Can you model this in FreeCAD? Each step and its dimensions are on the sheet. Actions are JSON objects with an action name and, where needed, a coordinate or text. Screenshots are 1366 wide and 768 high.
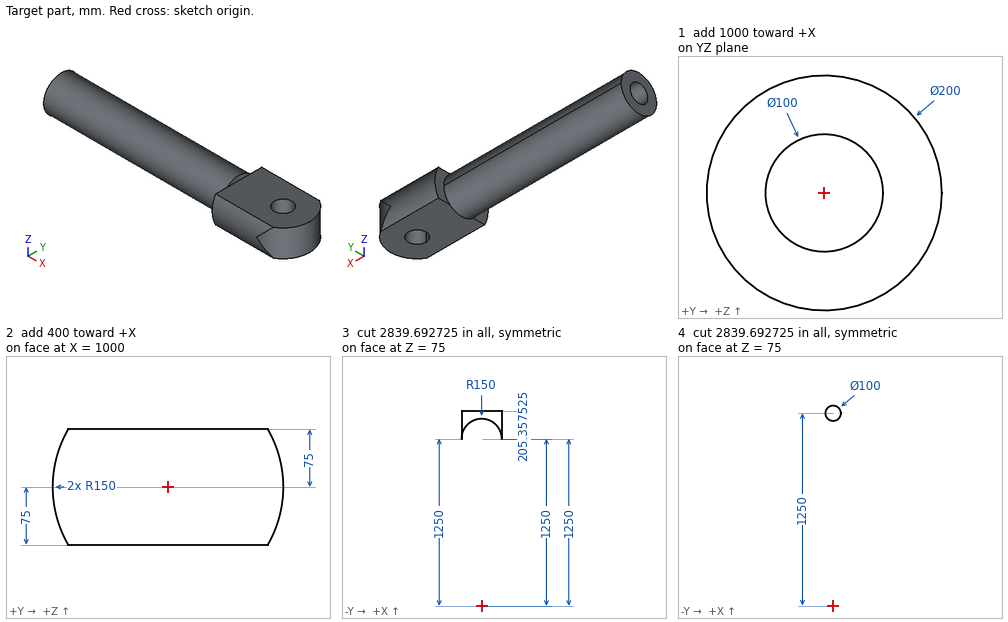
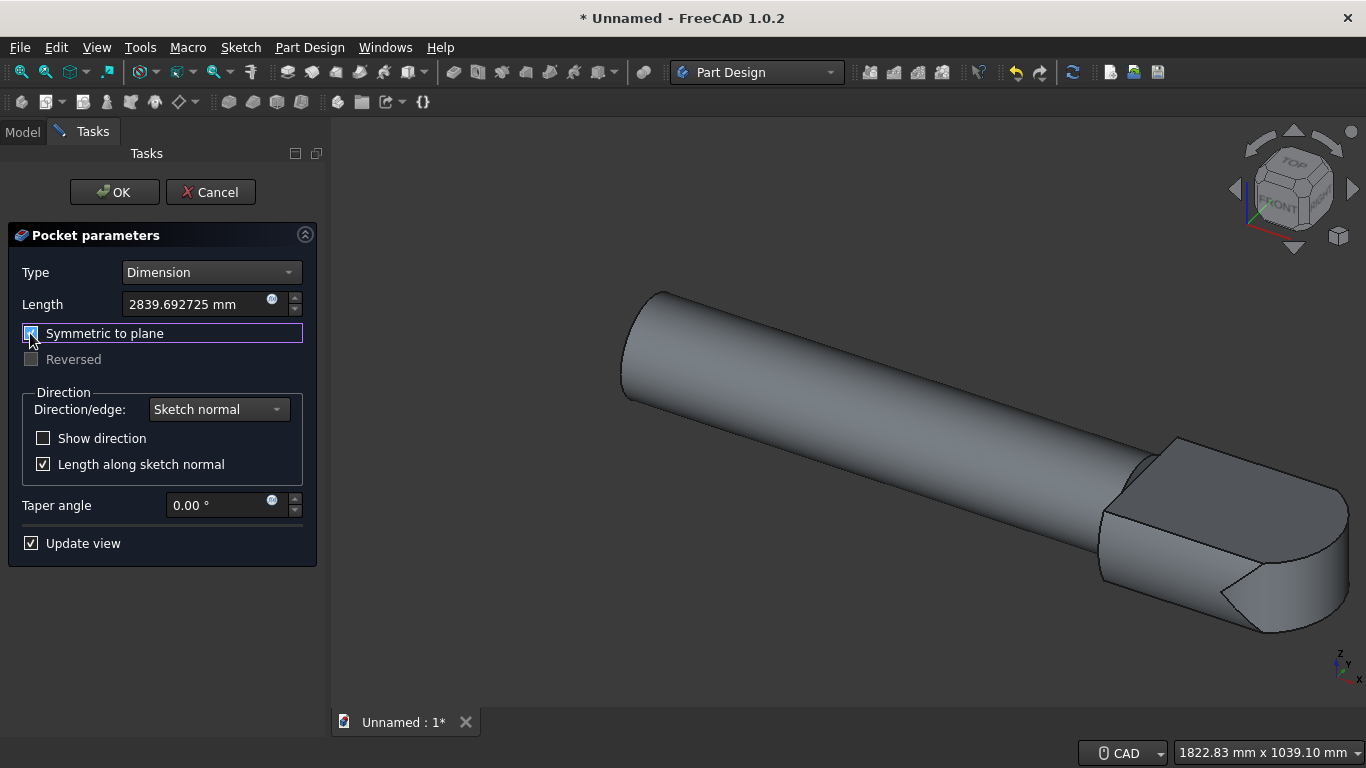
{"action": "left_click", "coordinate": [115, 192]}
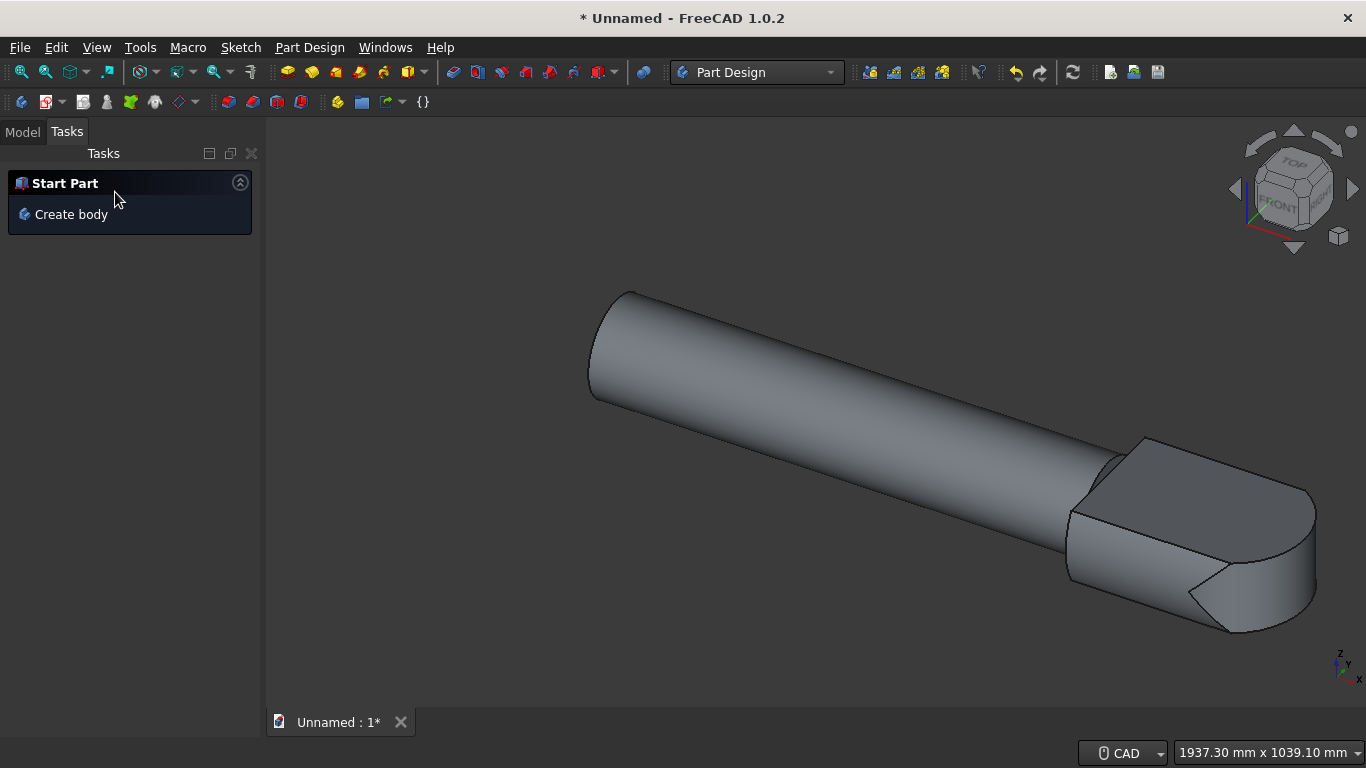
{"action": "left_click", "coordinate": [1207, 506]}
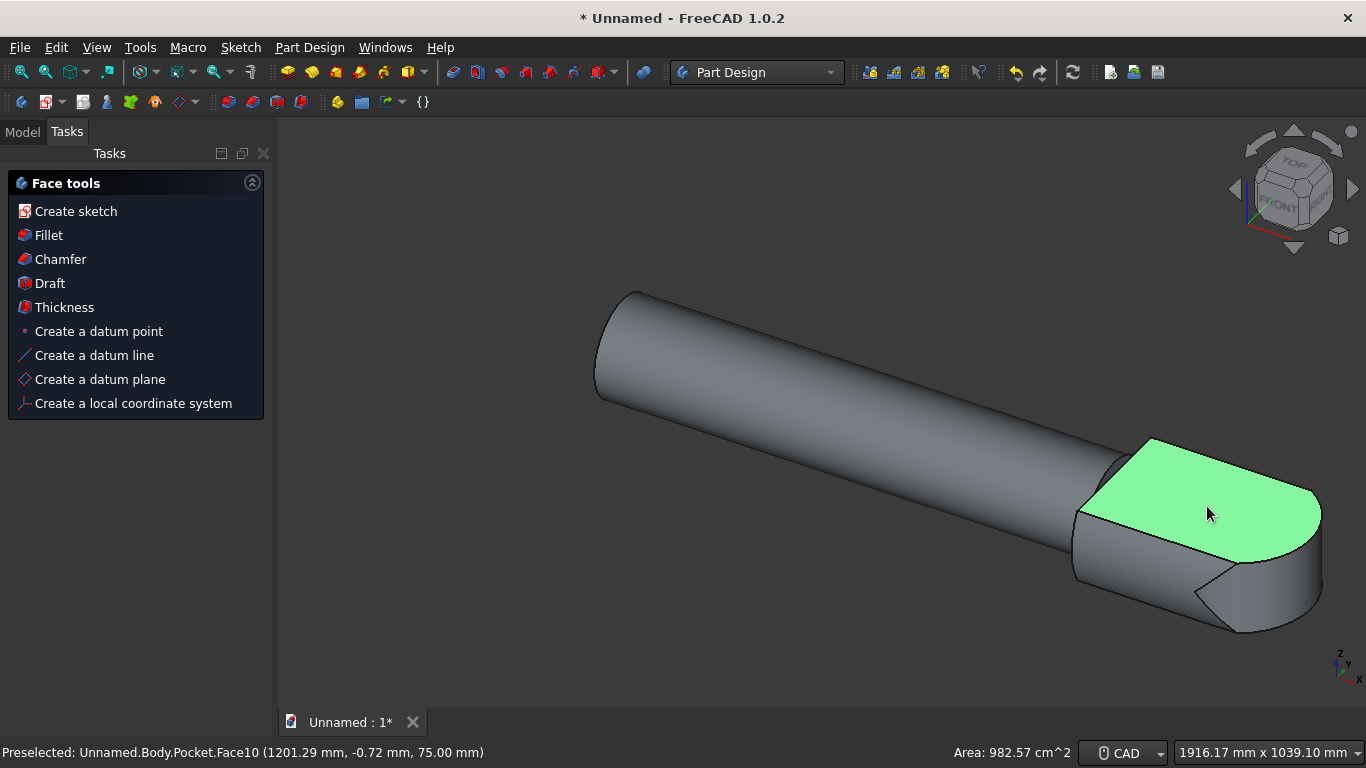
{"action": "left_click", "coordinate": [46, 102]}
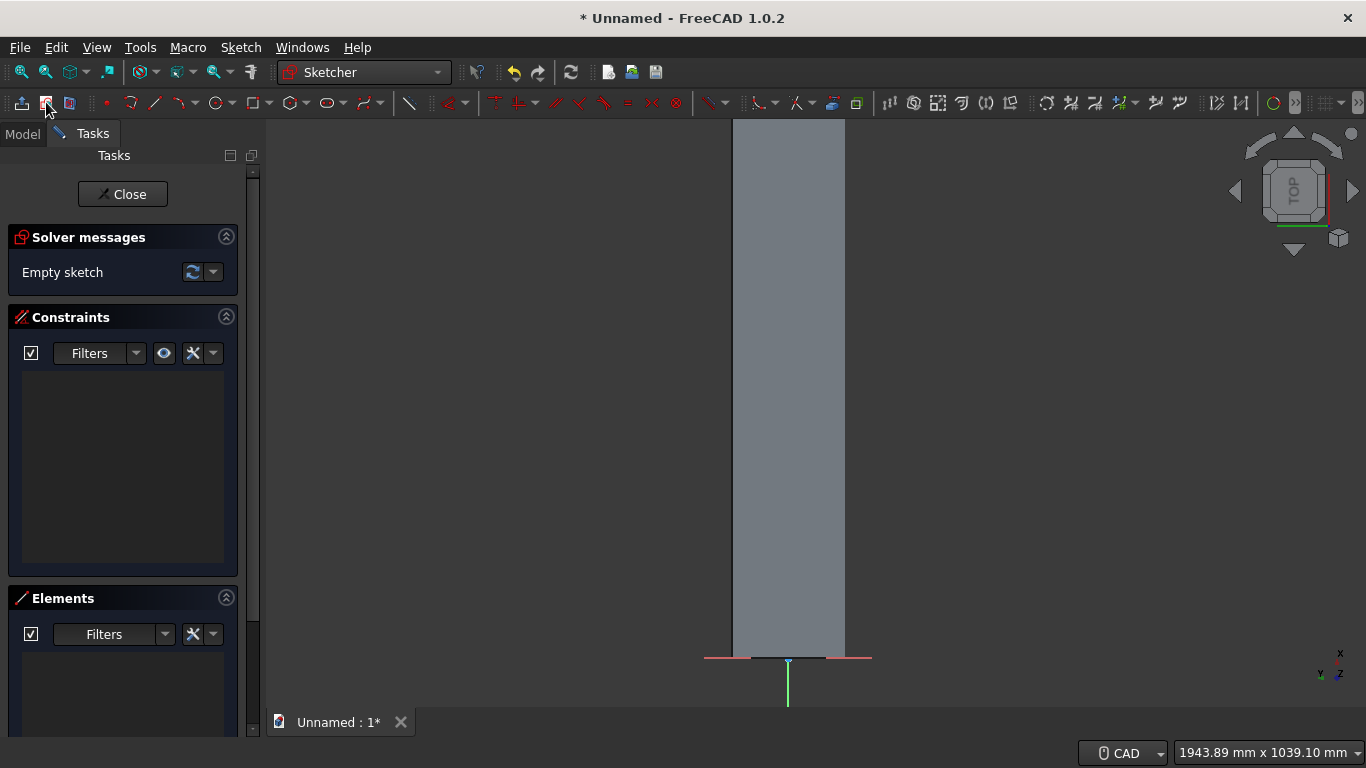
{"action": "left_click", "coordinate": [70, 104]}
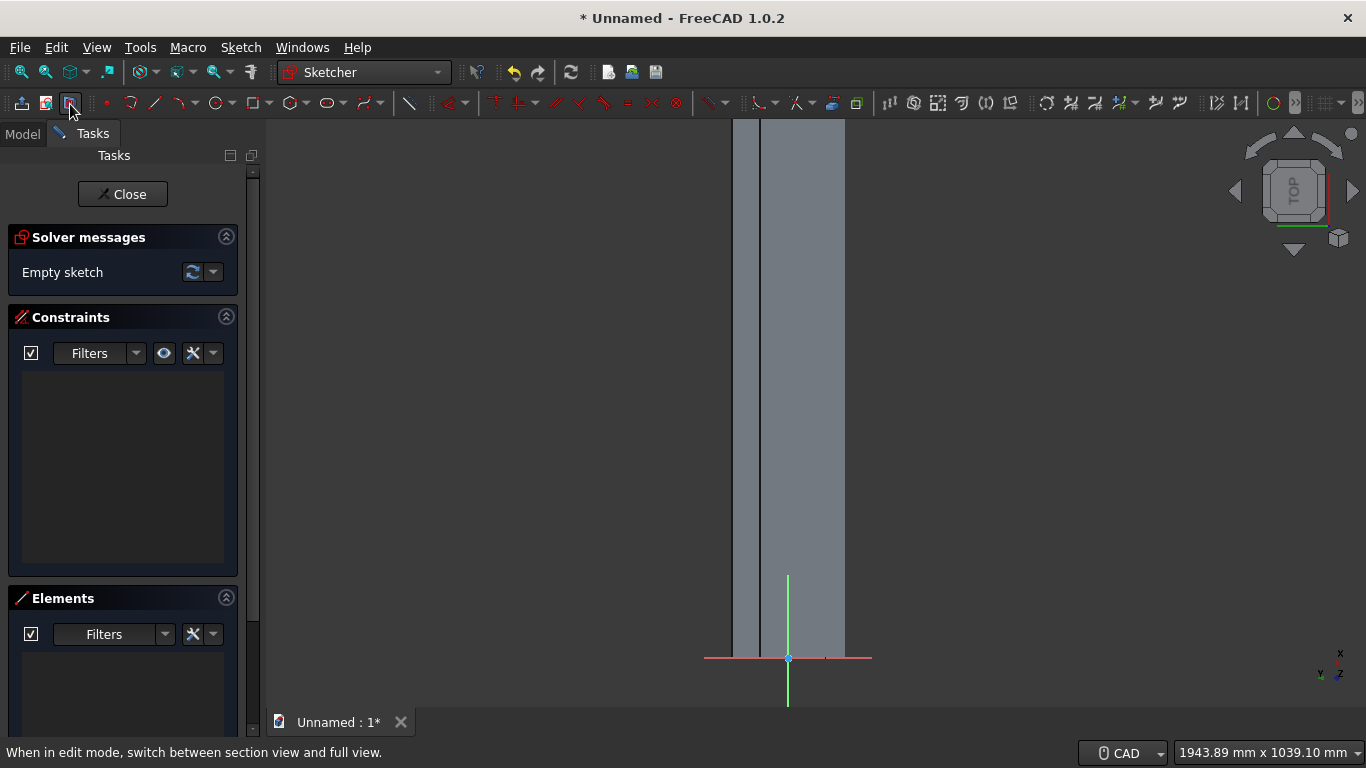
{"action": "scroll", "coordinate": [748, 413], "scroll_direction": "down", "scroll_amount": 5}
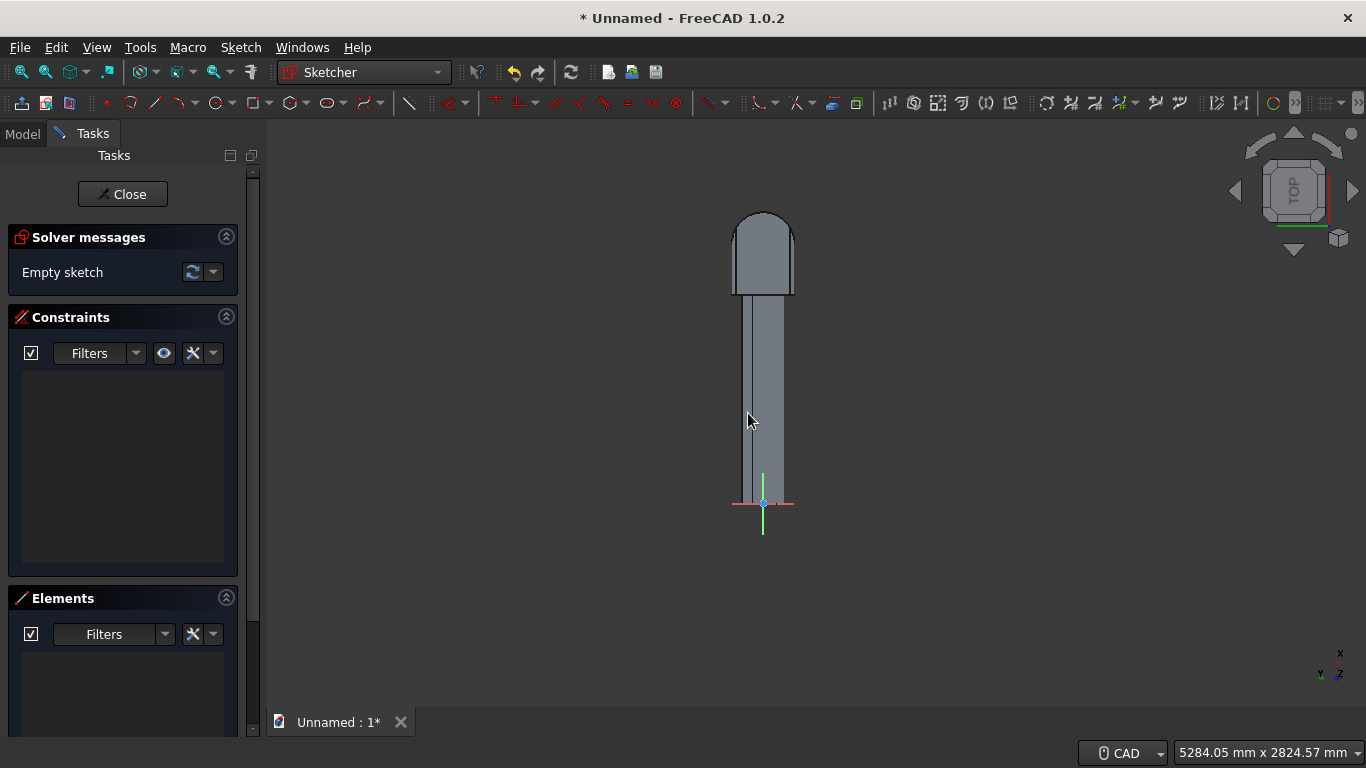
{"action": "scroll", "coordinate": [764, 232], "scroll_direction": "up", "scroll_amount": 14}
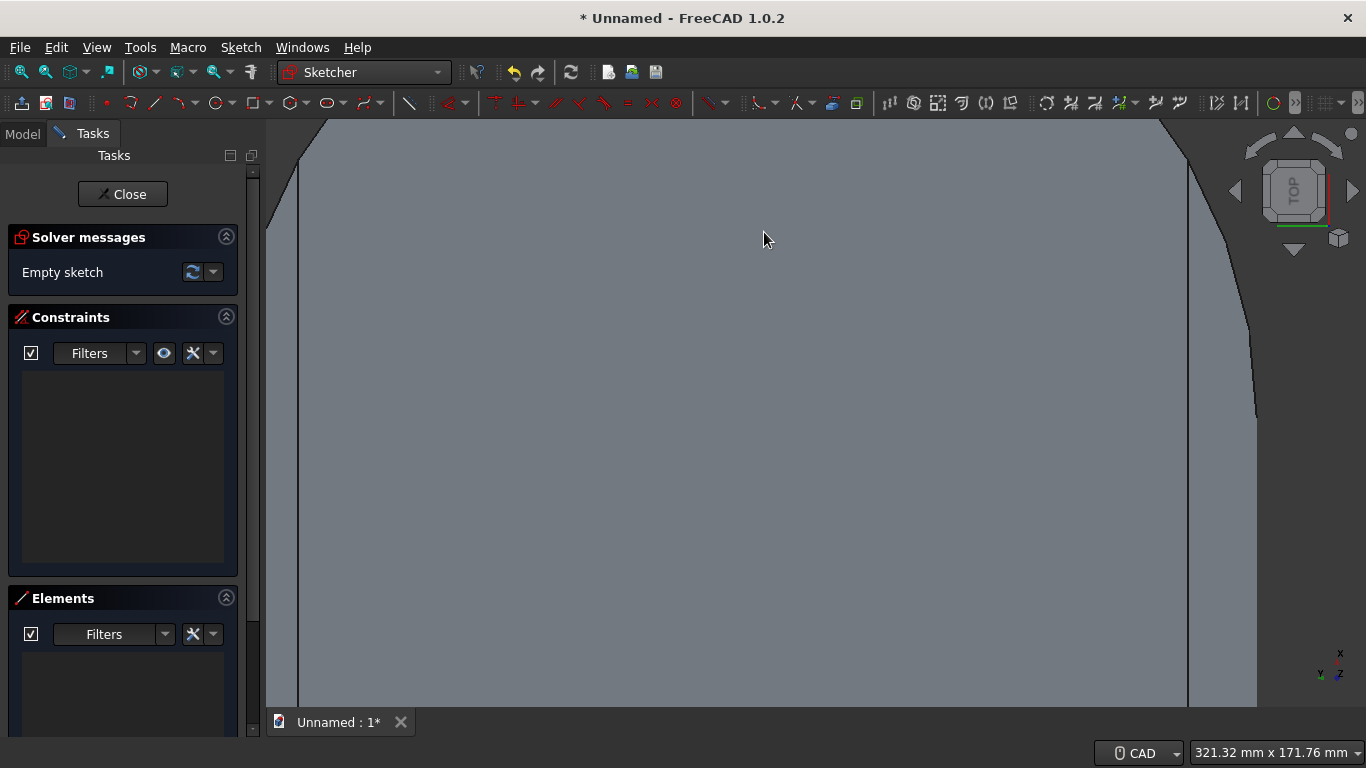
{"action": "left_click", "coordinate": [216, 104]}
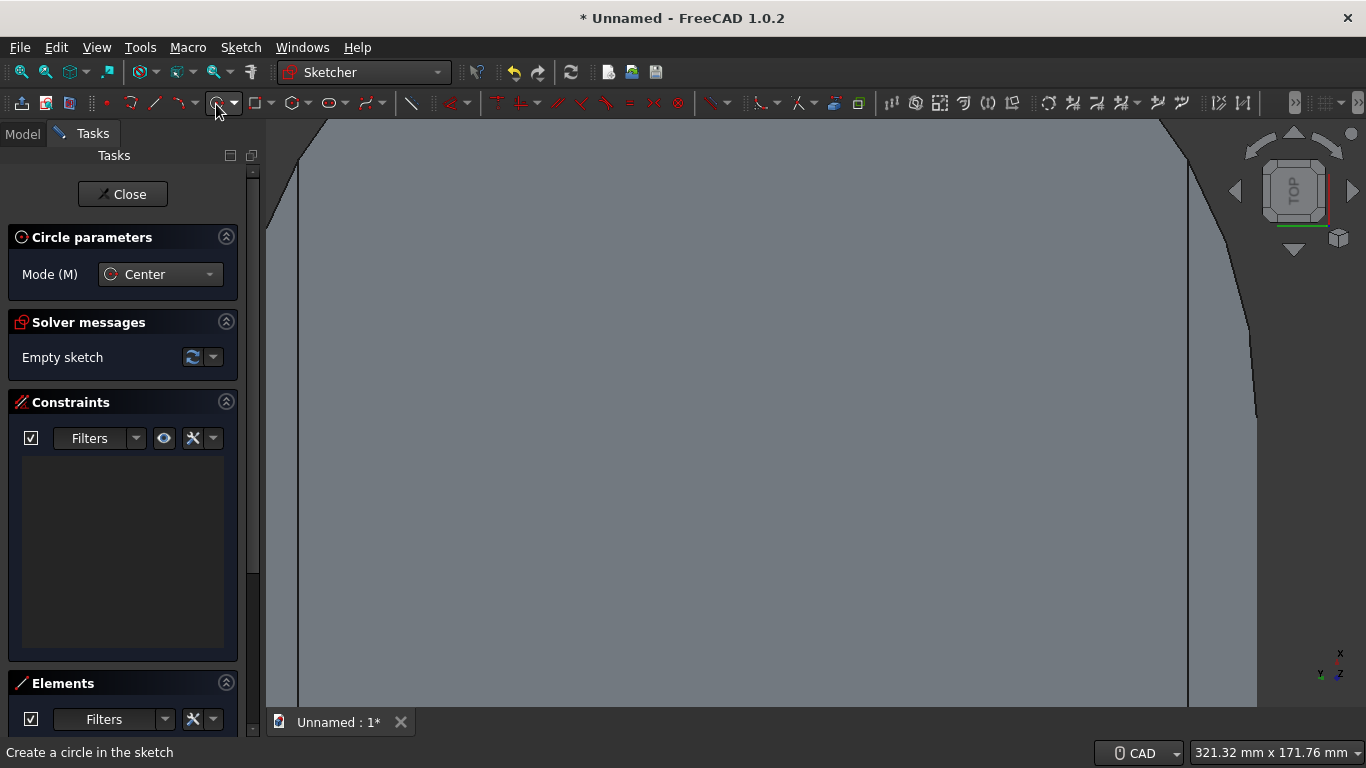
{"action": "left_click", "coordinate": [743, 417]}
{"action": "mouse_move", "coordinate": [864, 296]}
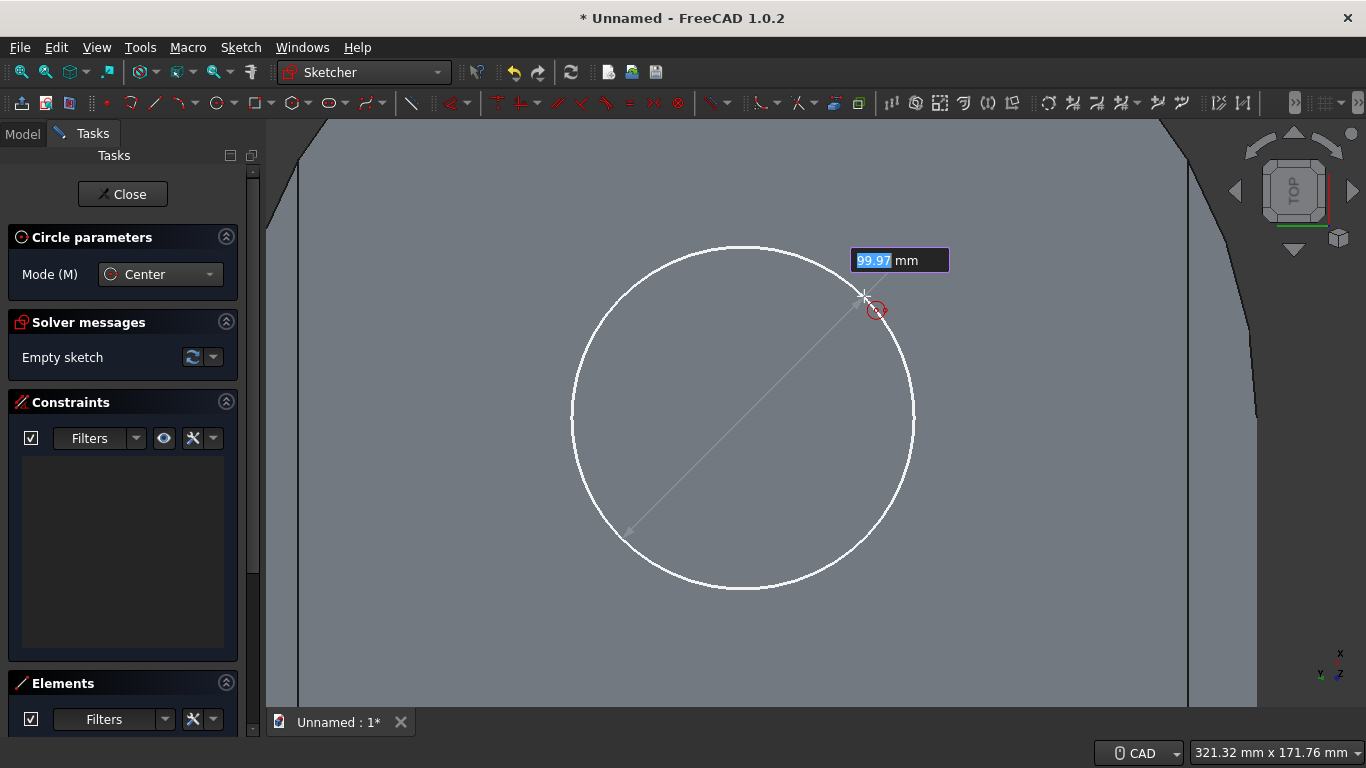
{"action": "type", "text": "100"}
{"action": "key", "text": "Return"}
{"action": "key", "text": "Escape"}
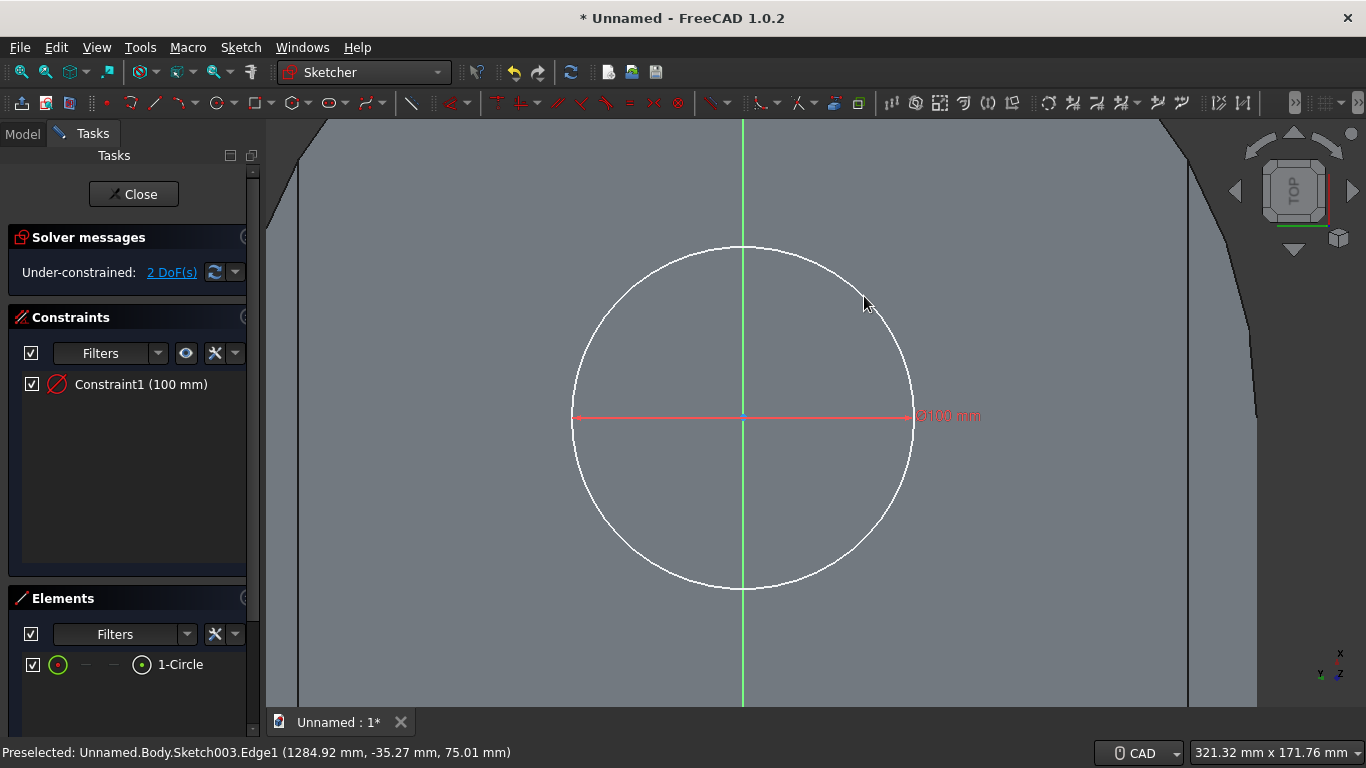
{"action": "left_click", "coordinate": [743, 418]}